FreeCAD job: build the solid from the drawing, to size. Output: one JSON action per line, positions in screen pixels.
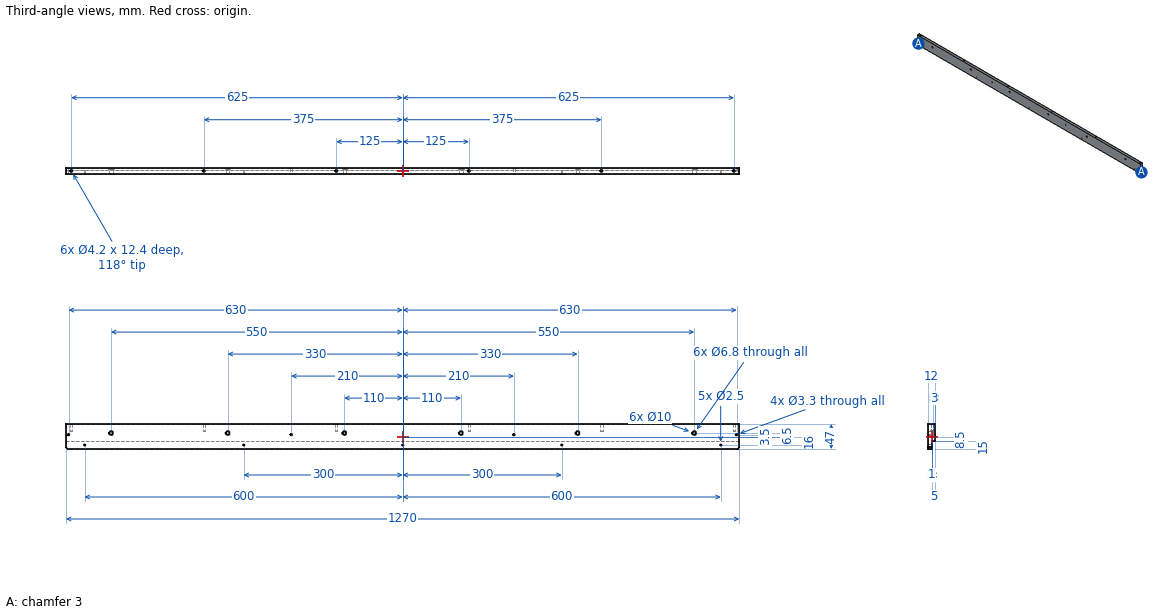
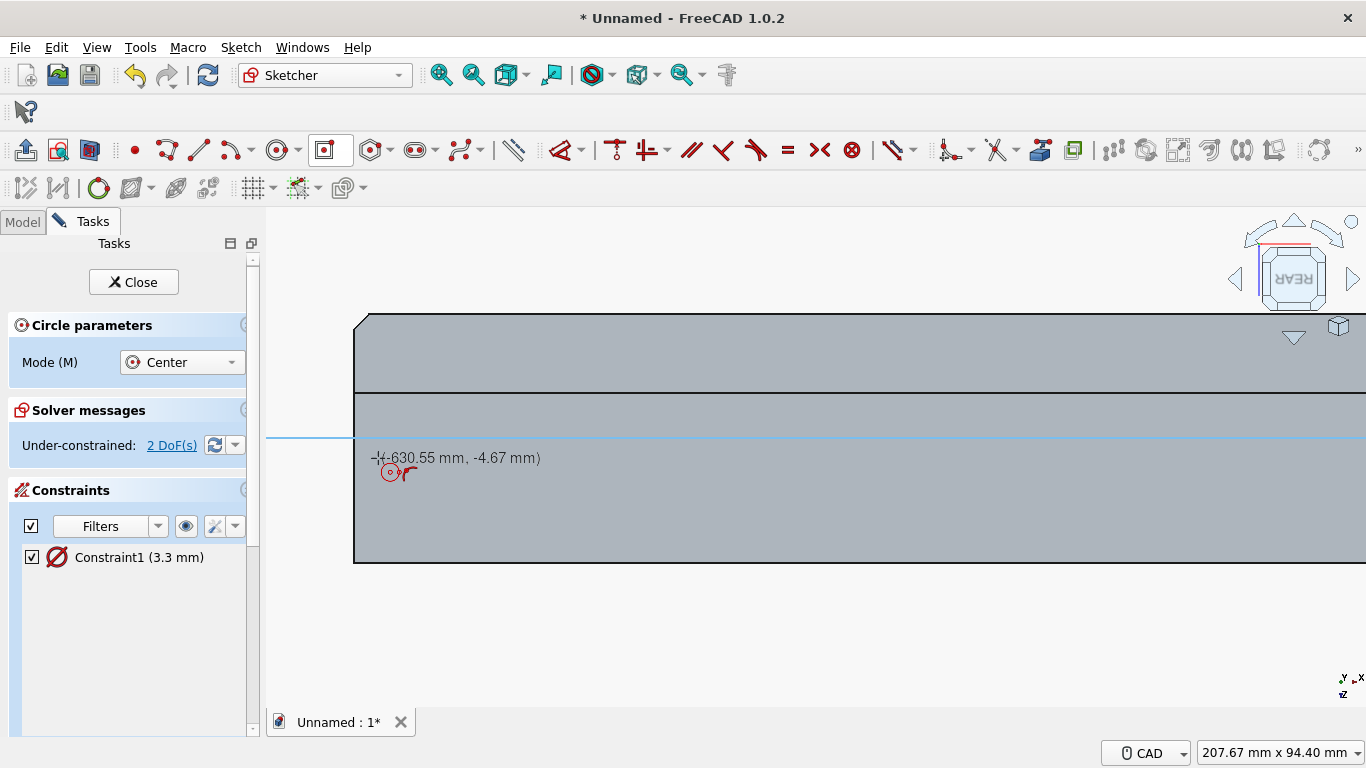
{"action": "left_click", "coordinate": [380, 457]}
{"action": "mouse_move", "coordinate": [386, 463]}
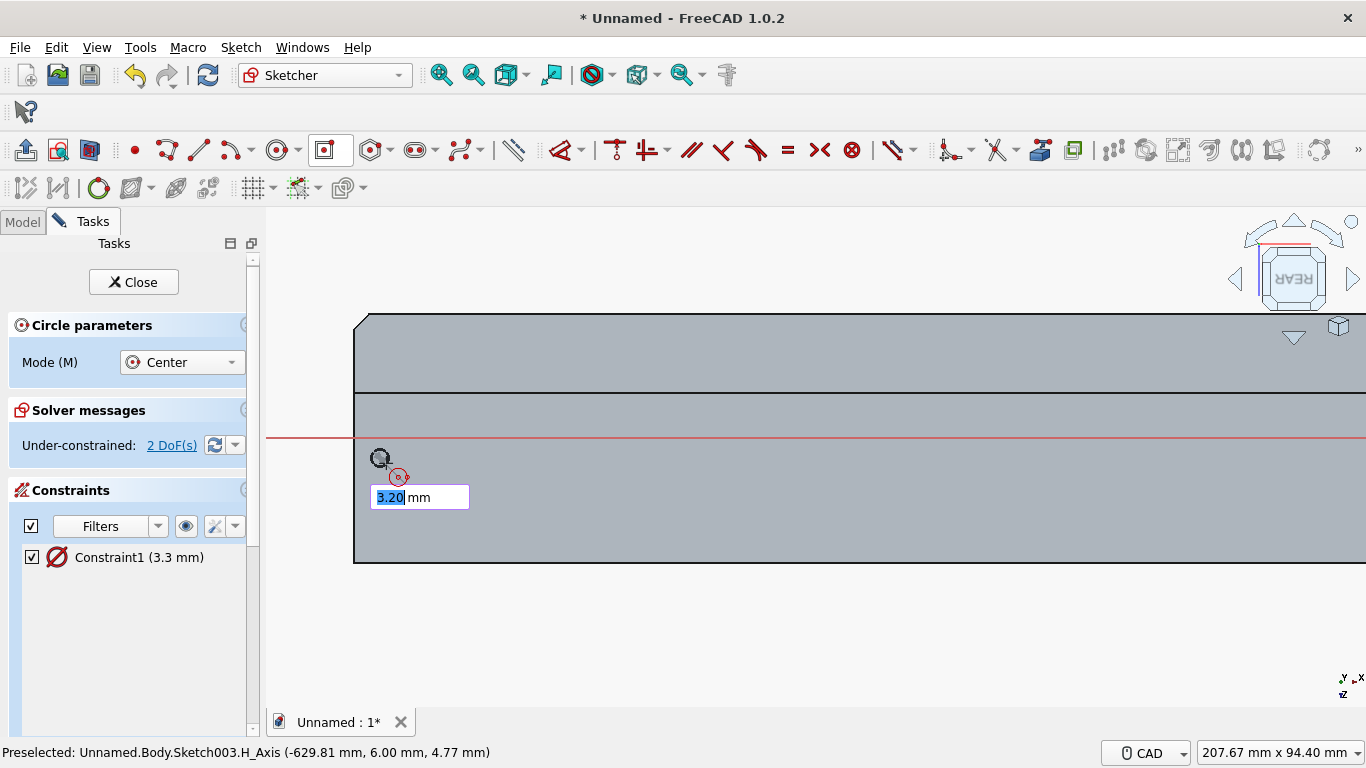
{"action": "type", "text": "3.3"}
{"action": "key", "text": "Return"}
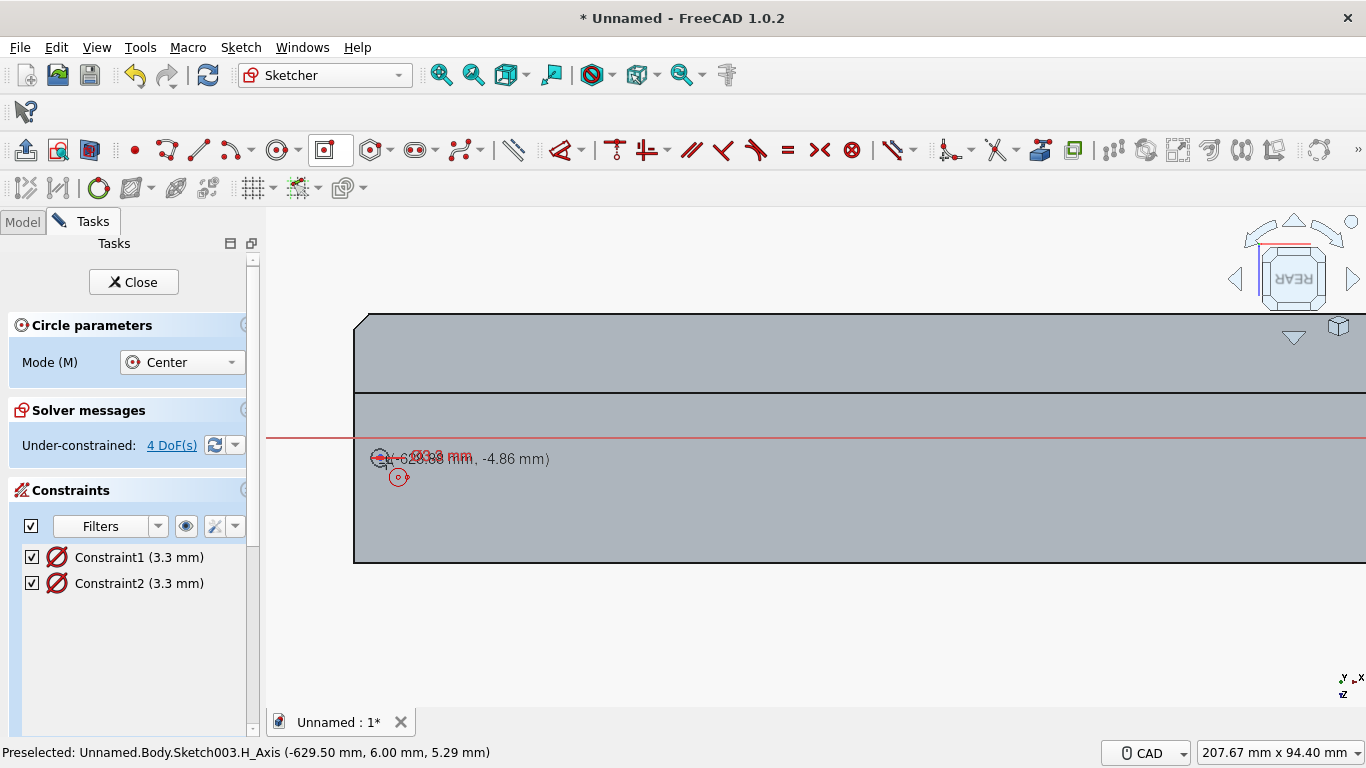
{"action": "scroll", "coordinate": [451, 458], "scroll_direction": "down", "scroll_amount": 12}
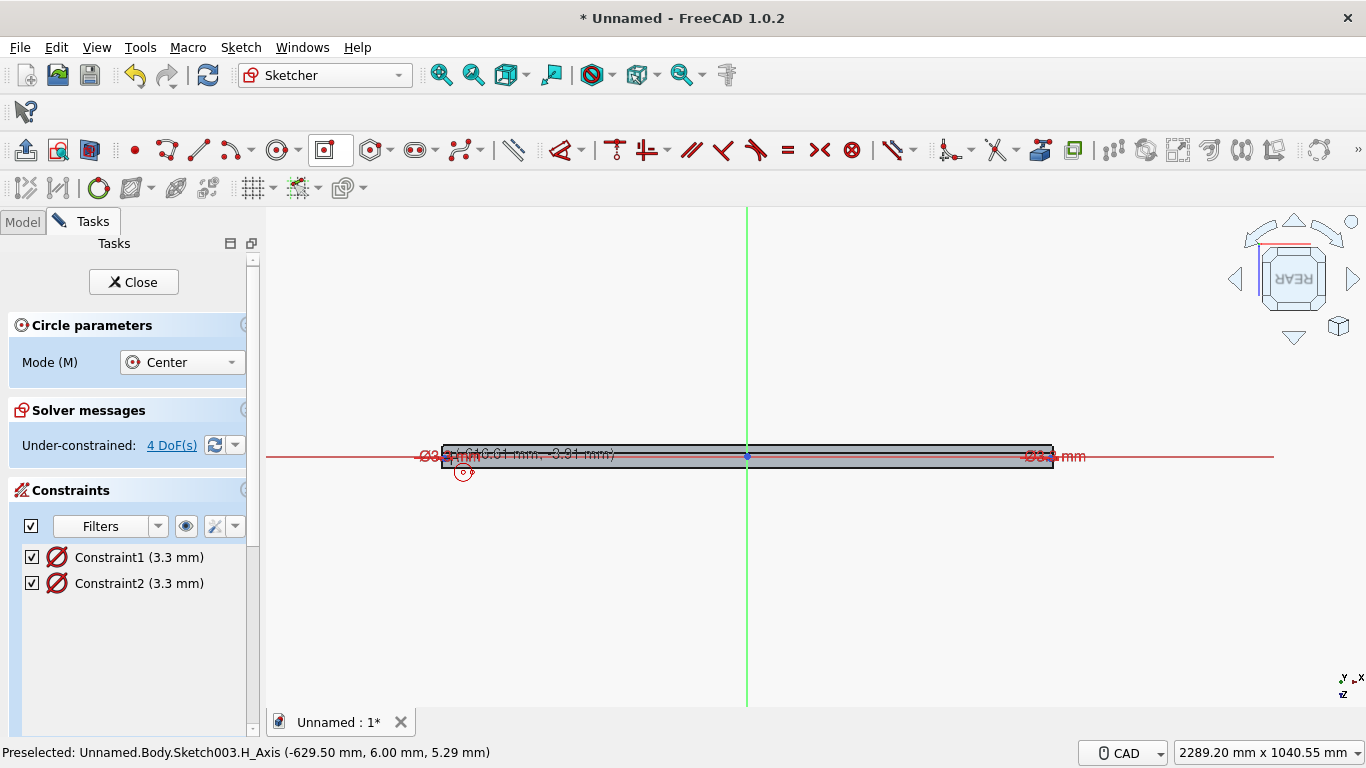
{"action": "scroll", "coordinate": [848, 458], "scroll_direction": "up", "scroll_amount": 17}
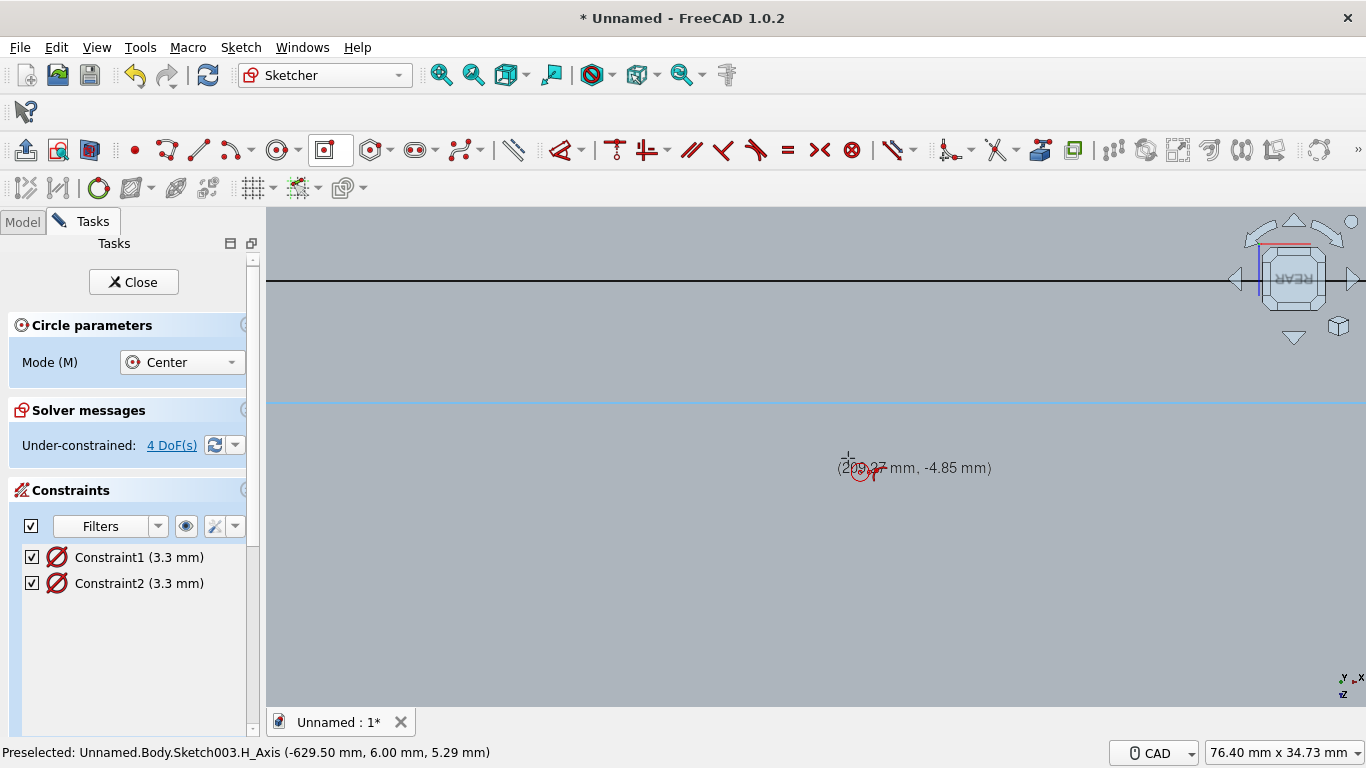
{"action": "scroll", "coordinate": [872, 458], "scroll_direction": "down", "scroll_amount": 16}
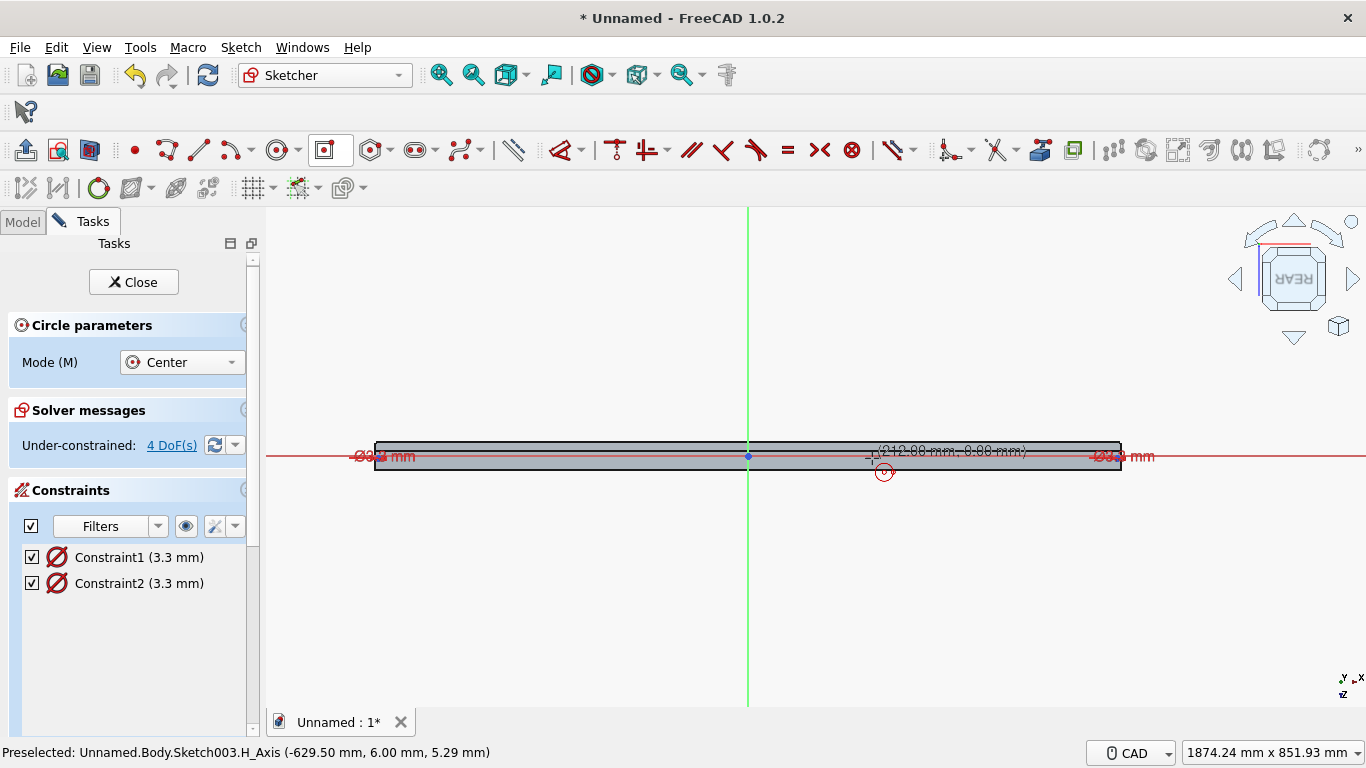
{"action": "scroll", "coordinate": [871, 458], "scroll_direction": "up", "scroll_amount": 11}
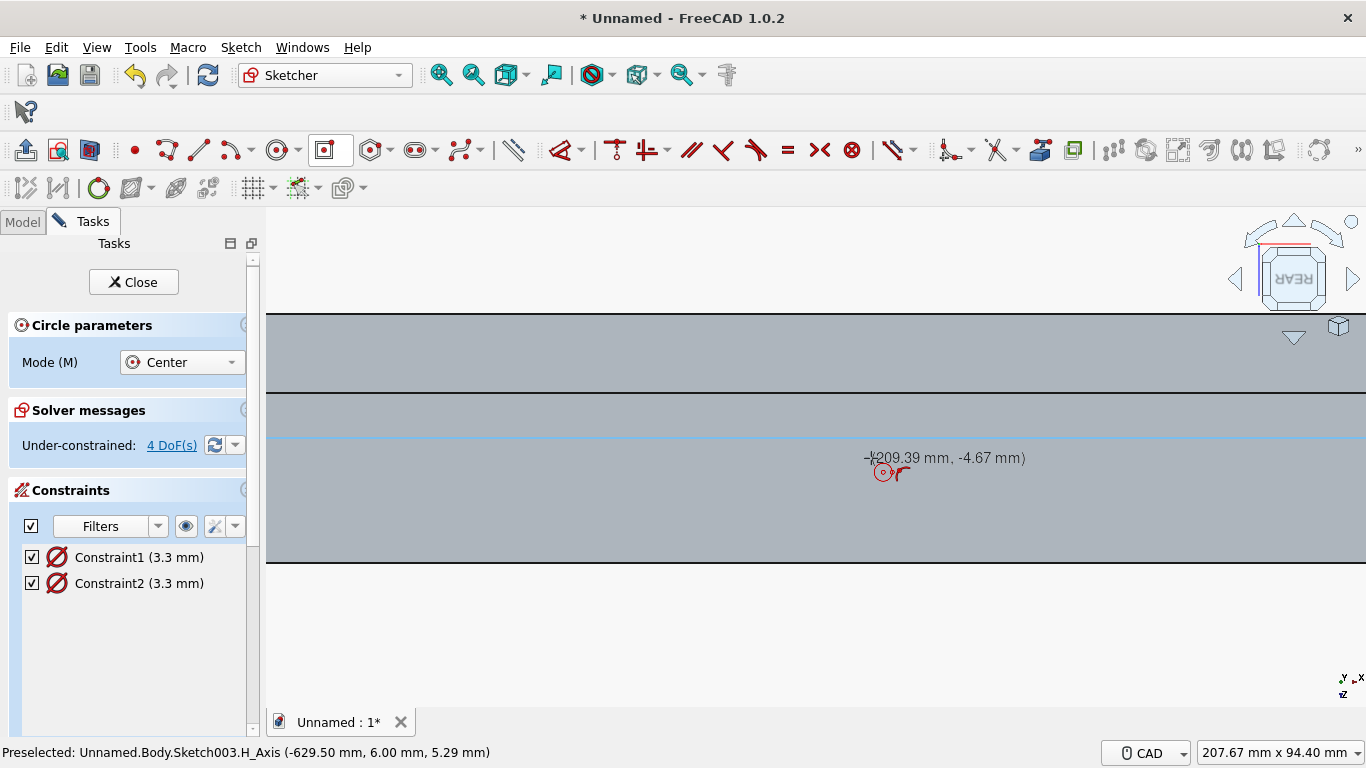
{"action": "left_click", "coordinate": [870, 457]}
{"action": "mouse_move", "coordinate": [876, 463]}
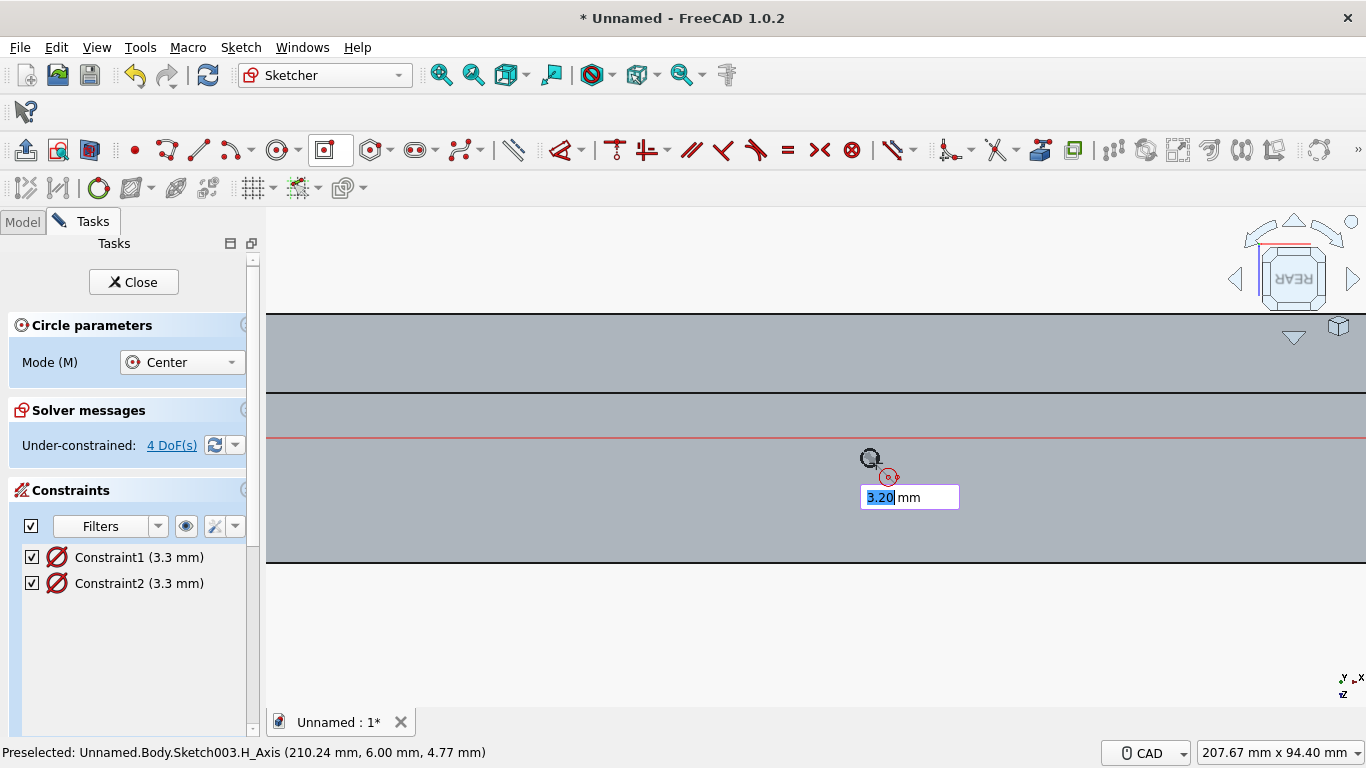
{"action": "type", "text": "3.3"}
{"action": "key", "text": "Return"}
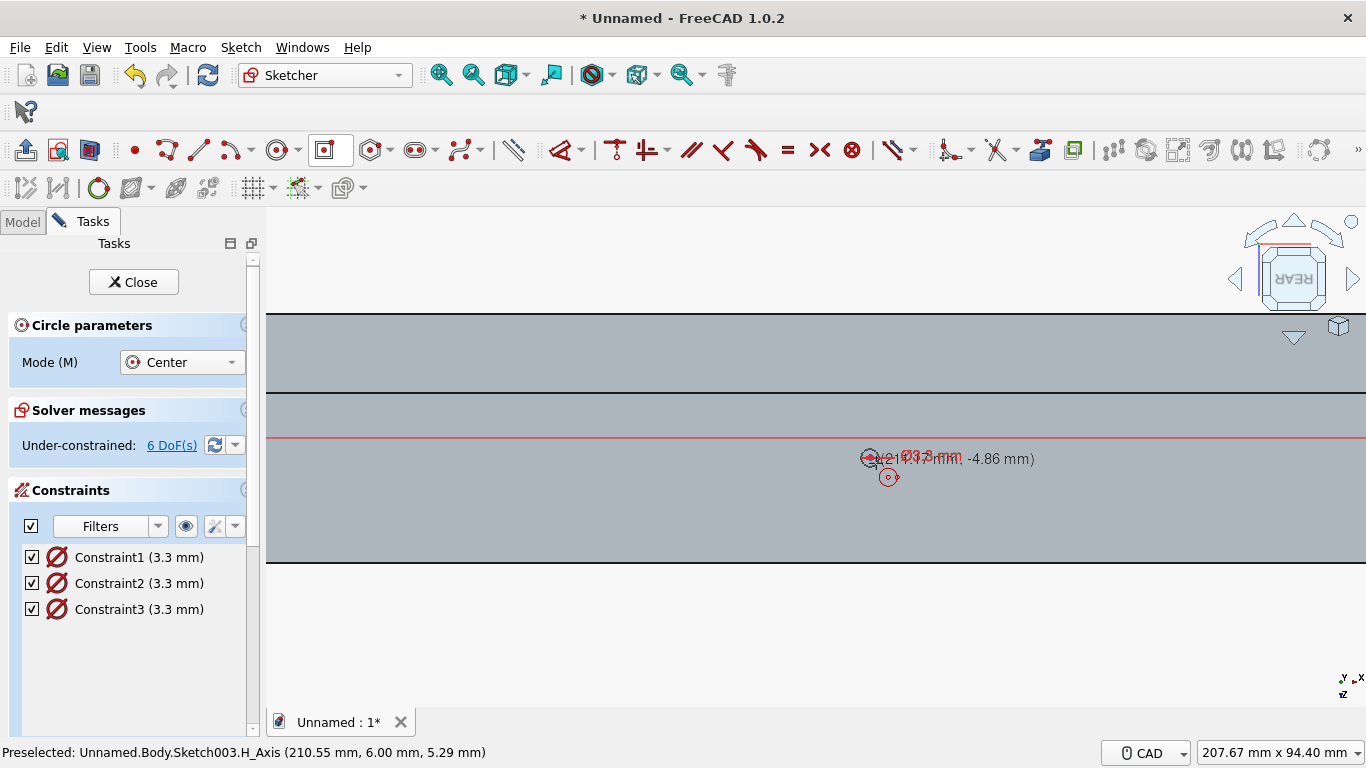
{"action": "scroll", "coordinate": [846, 458], "scroll_direction": "down", "scroll_amount": 12}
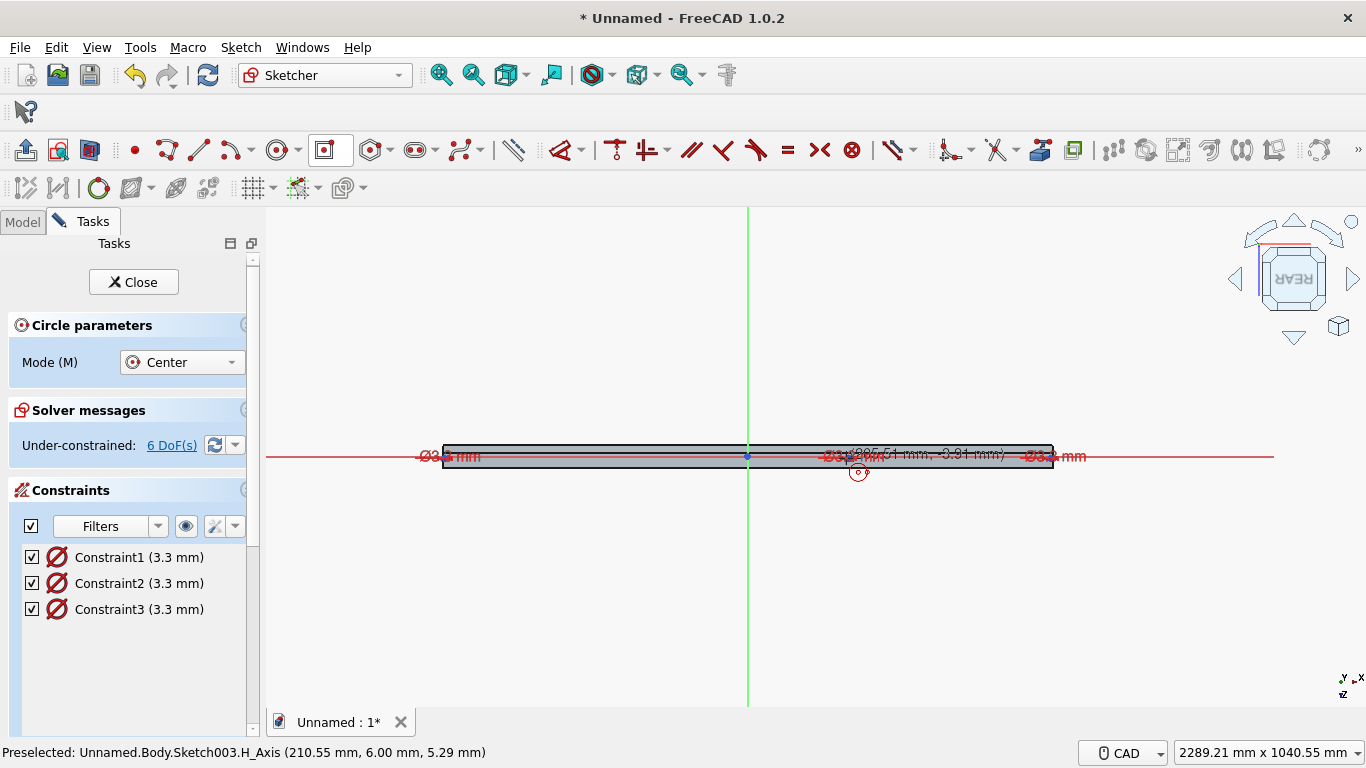
{"action": "scroll", "coordinate": [647, 458], "scroll_direction": "up", "scroll_amount": 17}